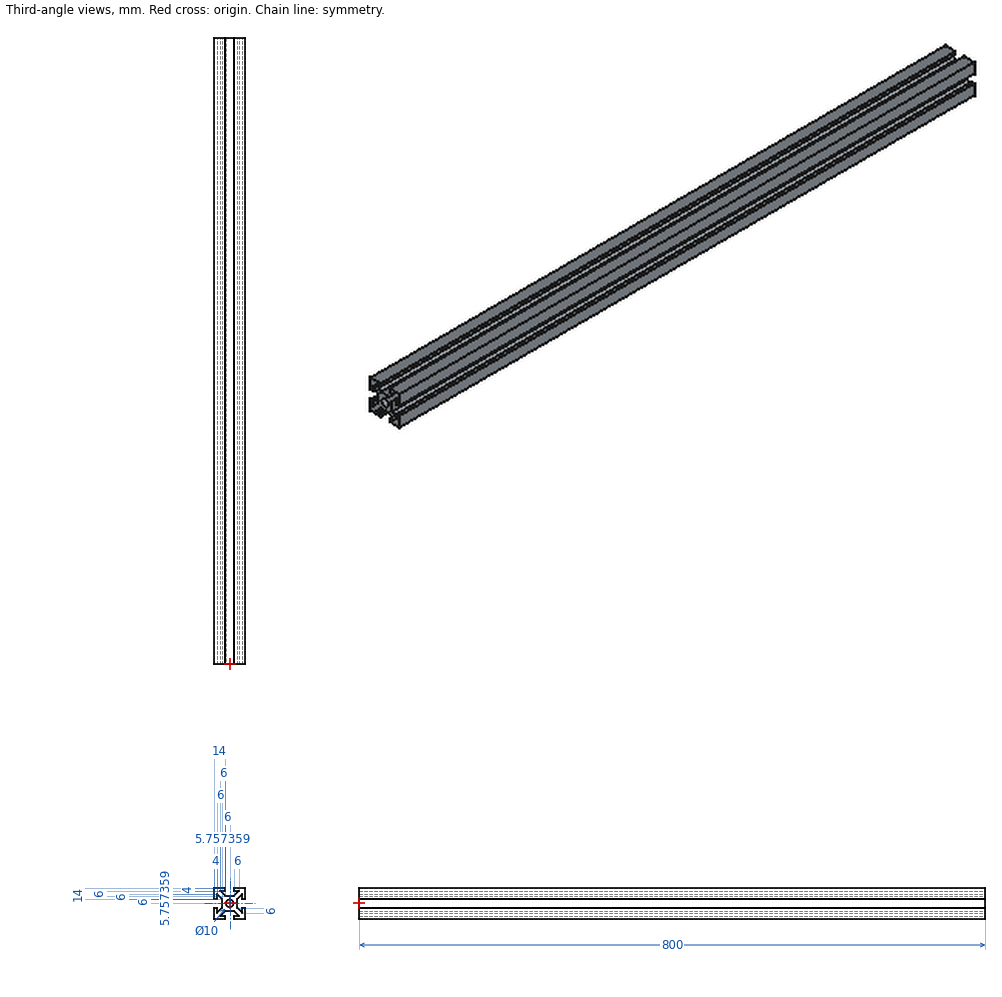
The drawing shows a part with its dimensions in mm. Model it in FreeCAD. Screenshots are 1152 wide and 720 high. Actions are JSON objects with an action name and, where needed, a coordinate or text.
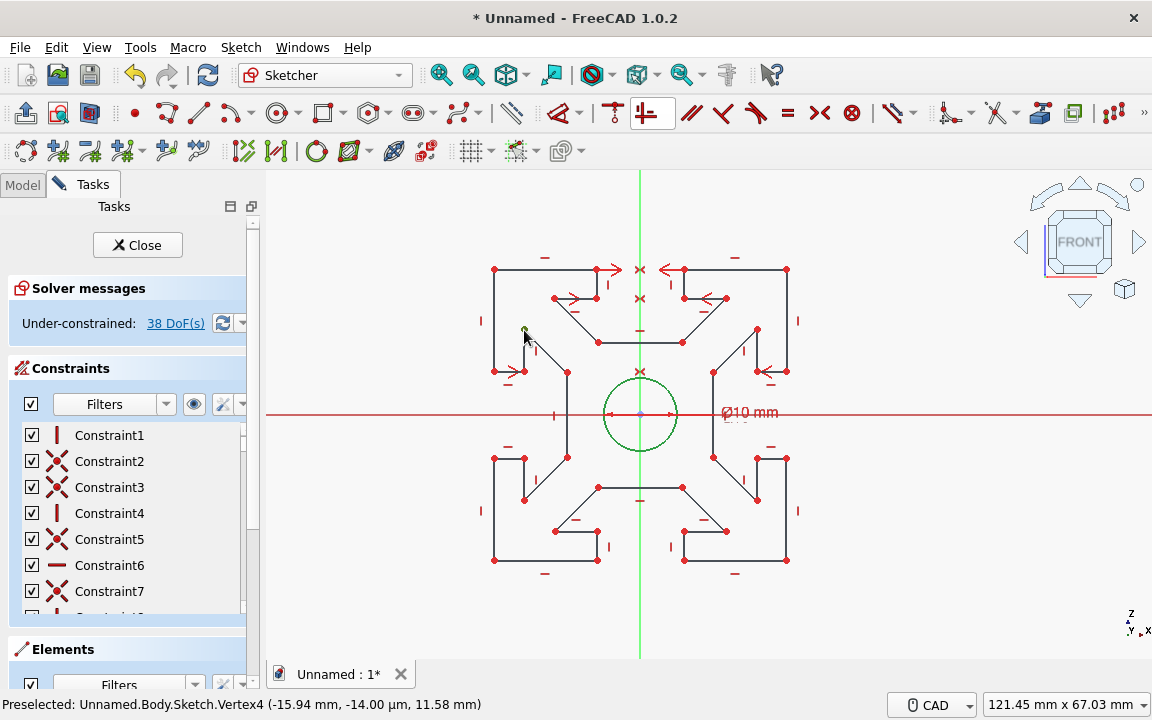
{"action": "left_click", "coordinate": [757, 330]}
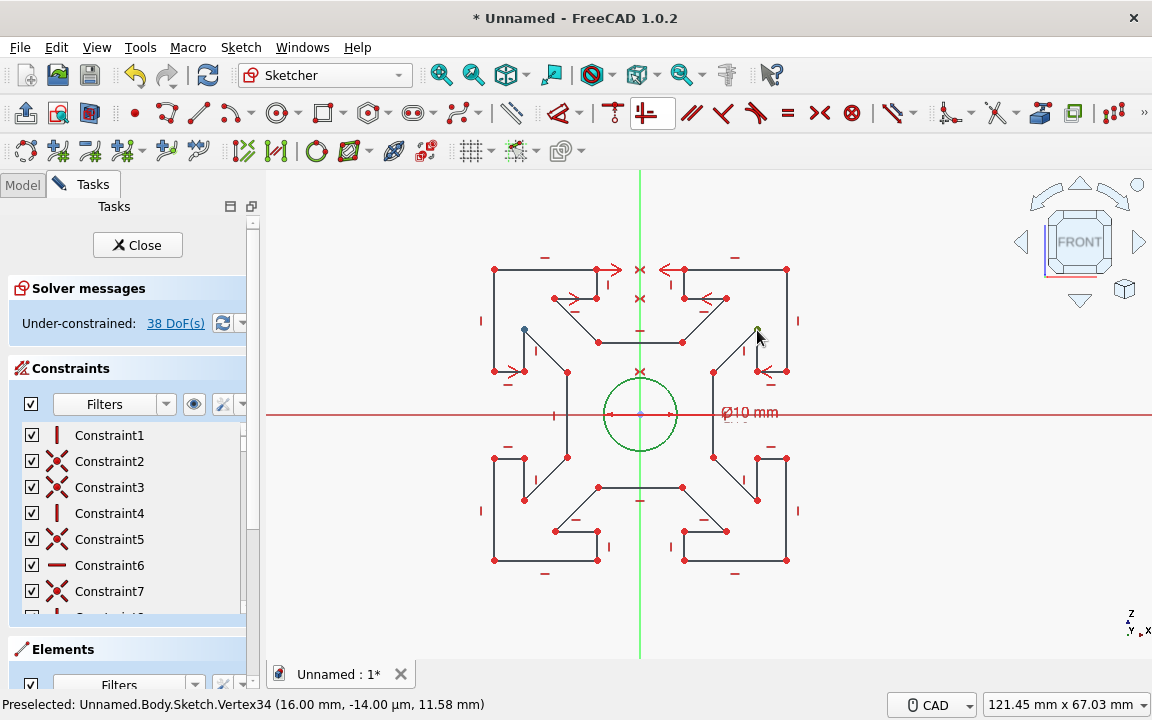
{"action": "left_click", "coordinate": [640, 600]}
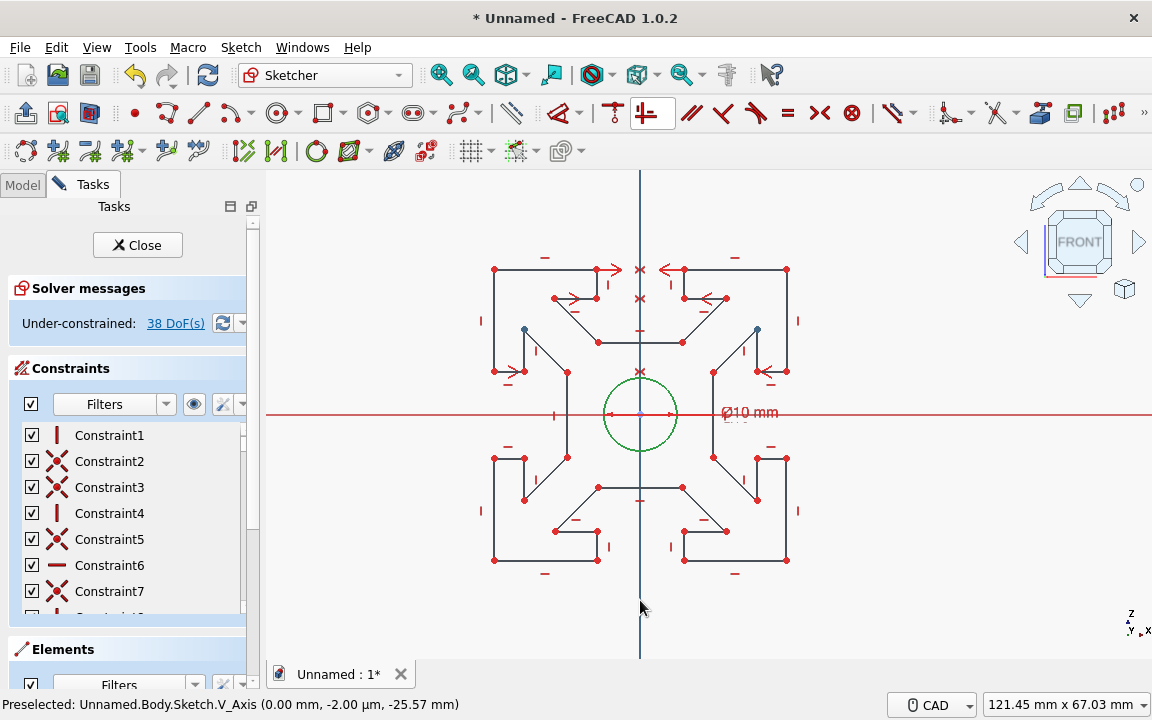
{"action": "key", "text": "s"}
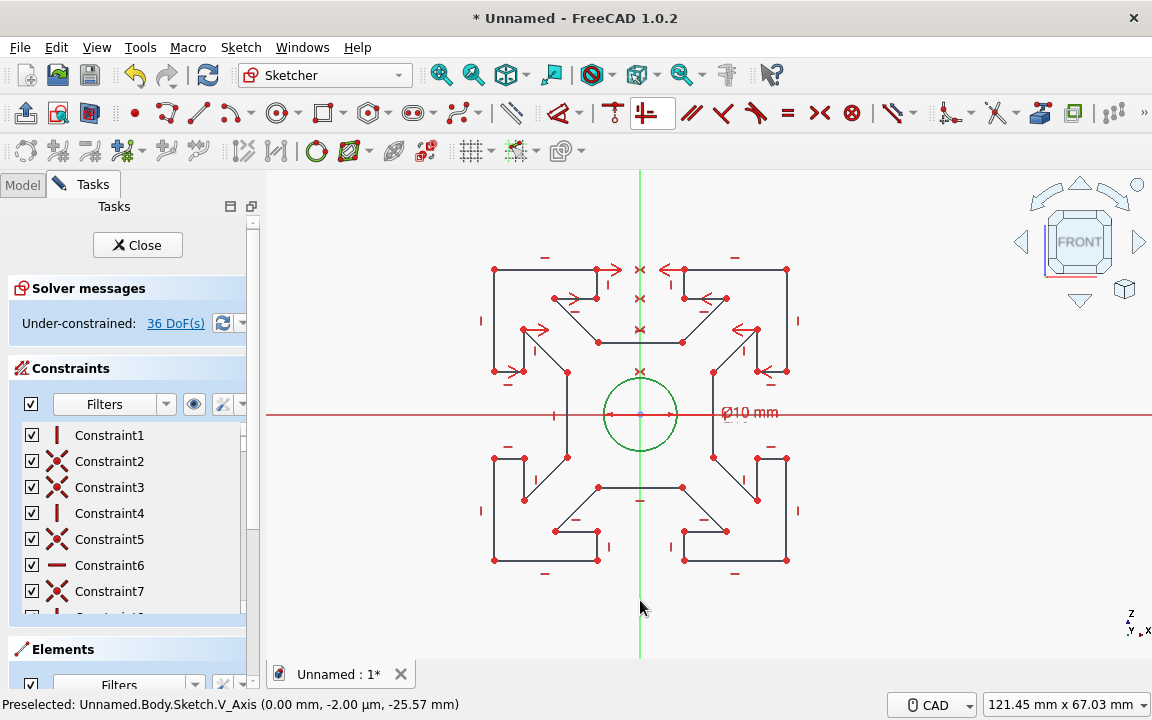
{"action": "left_click", "coordinate": [567, 373]}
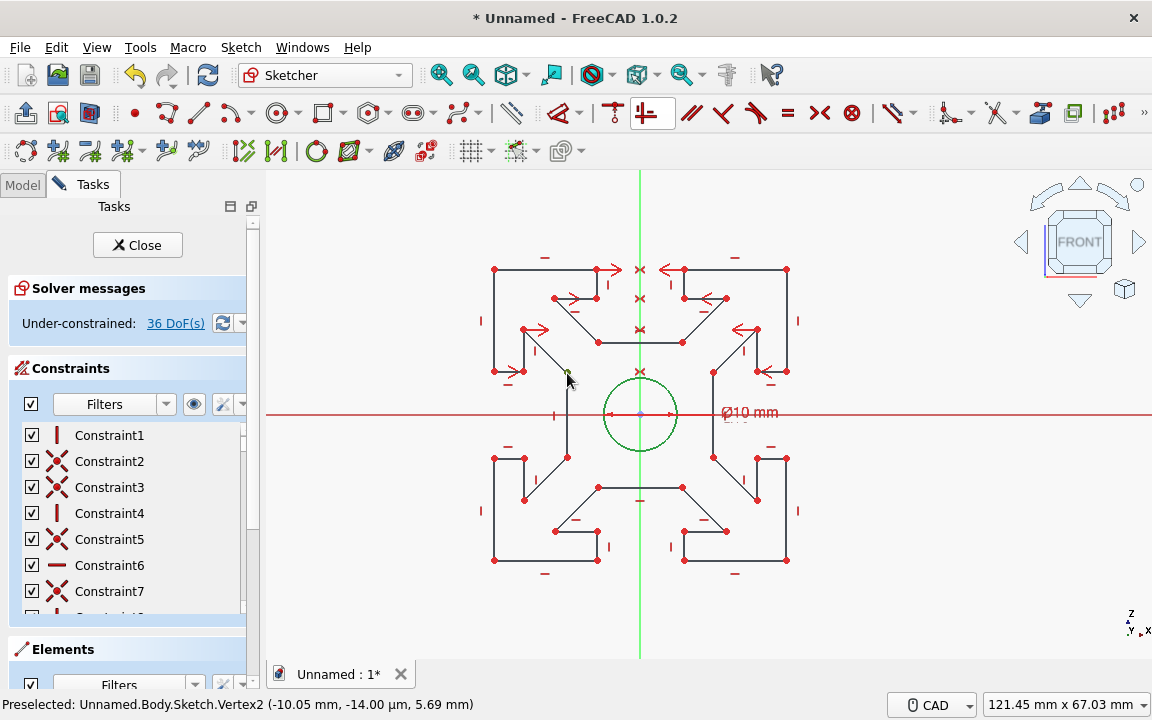
{"action": "left_click", "coordinate": [713, 373]}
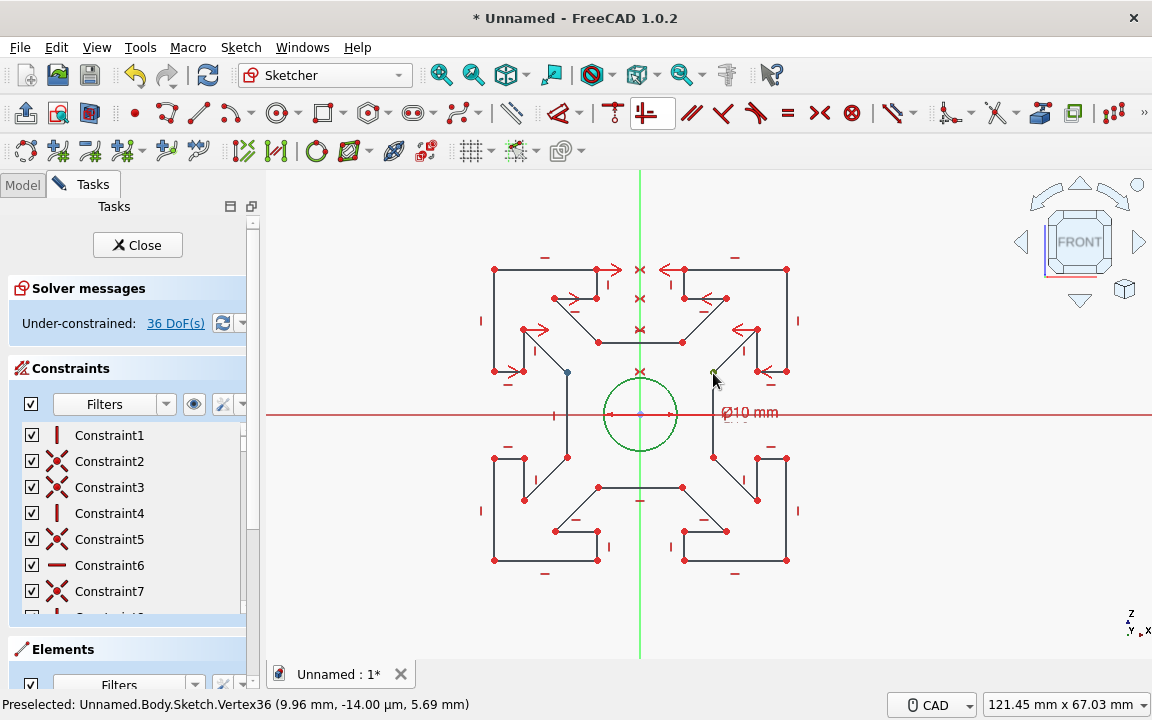
{"action": "left_click", "coordinate": [640, 600]}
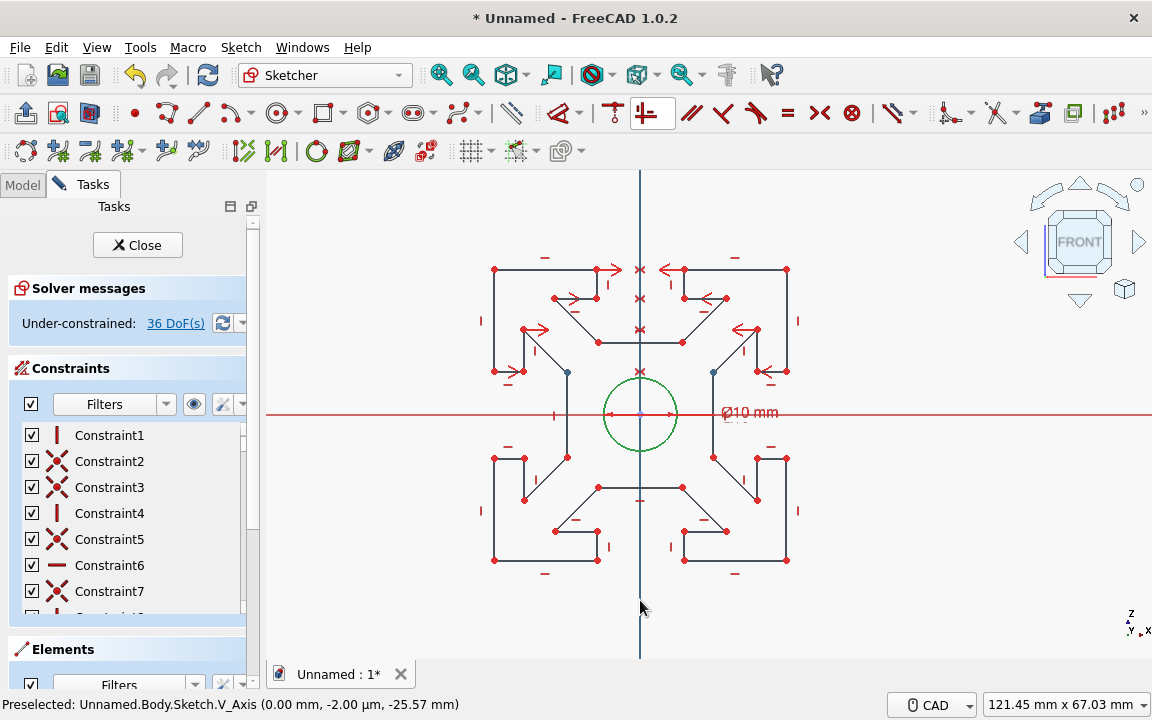
{"action": "left_click", "coordinate": [820, 114]}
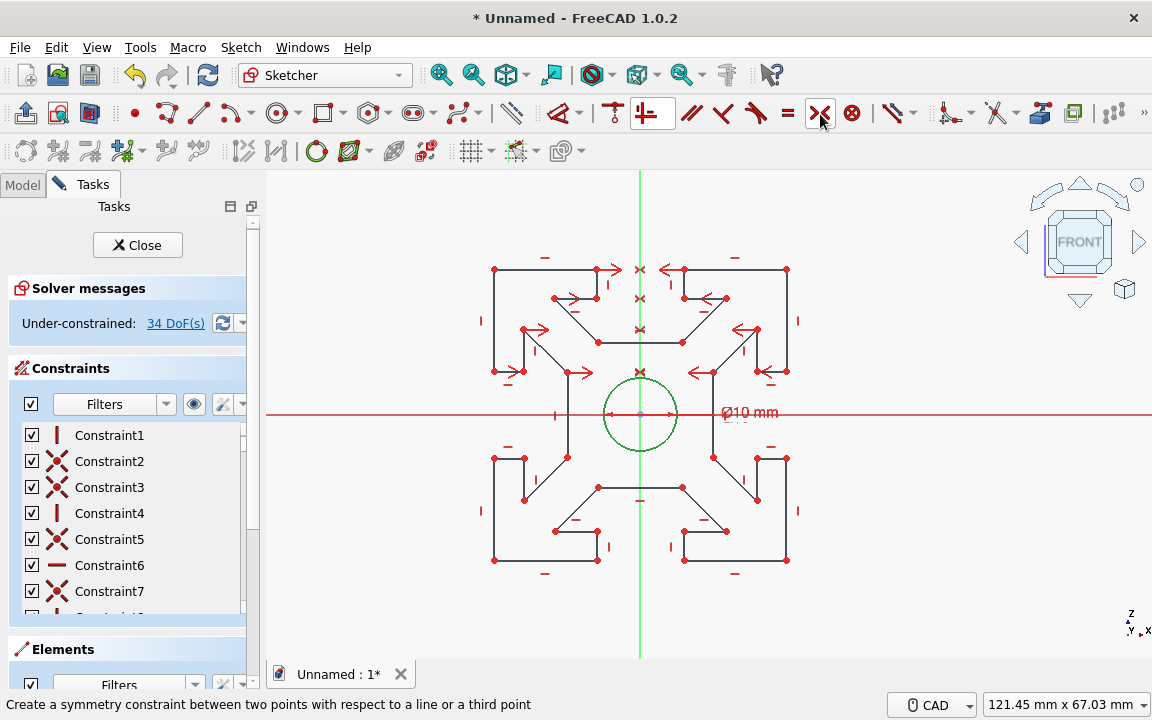
{"action": "left_click", "coordinate": [757, 330]}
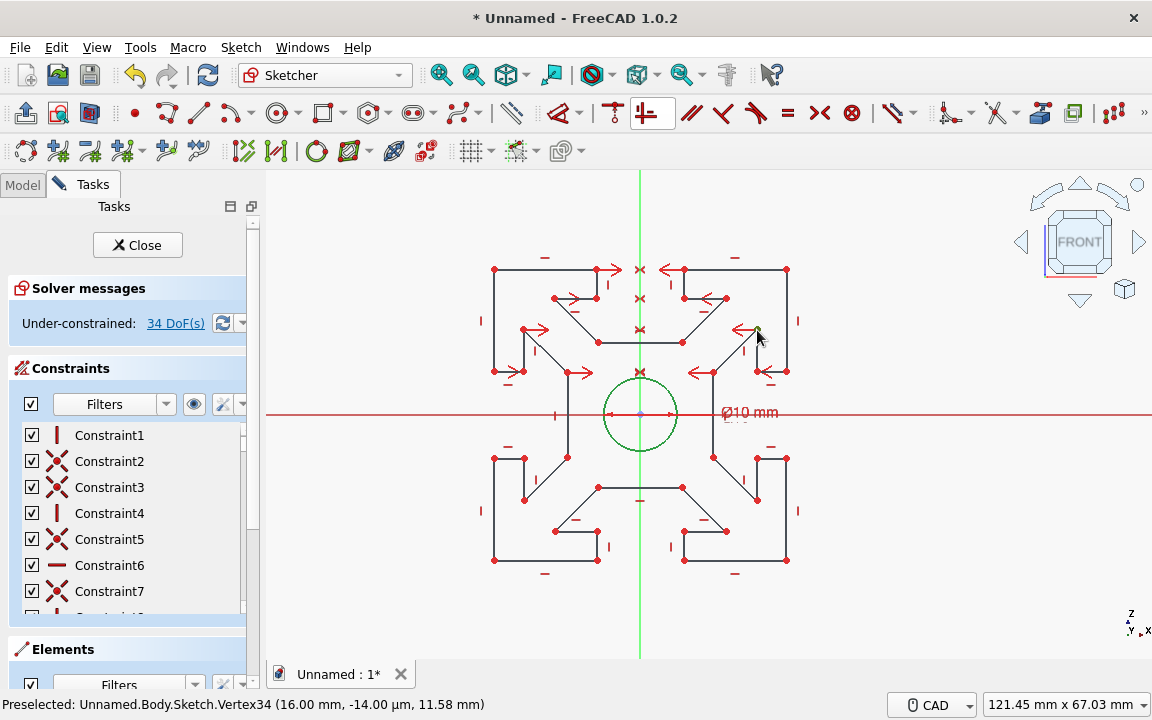
{"action": "left_click", "coordinate": [757, 501]}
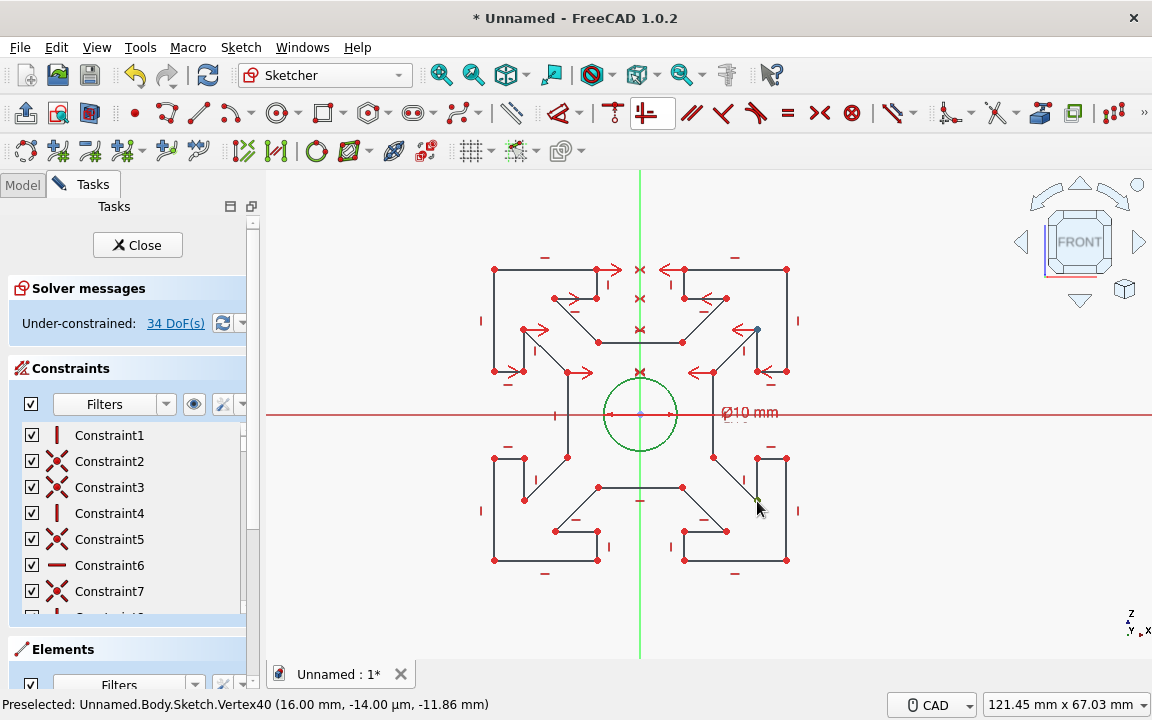
{"action": "left_click", "coordinate": [344, 414]}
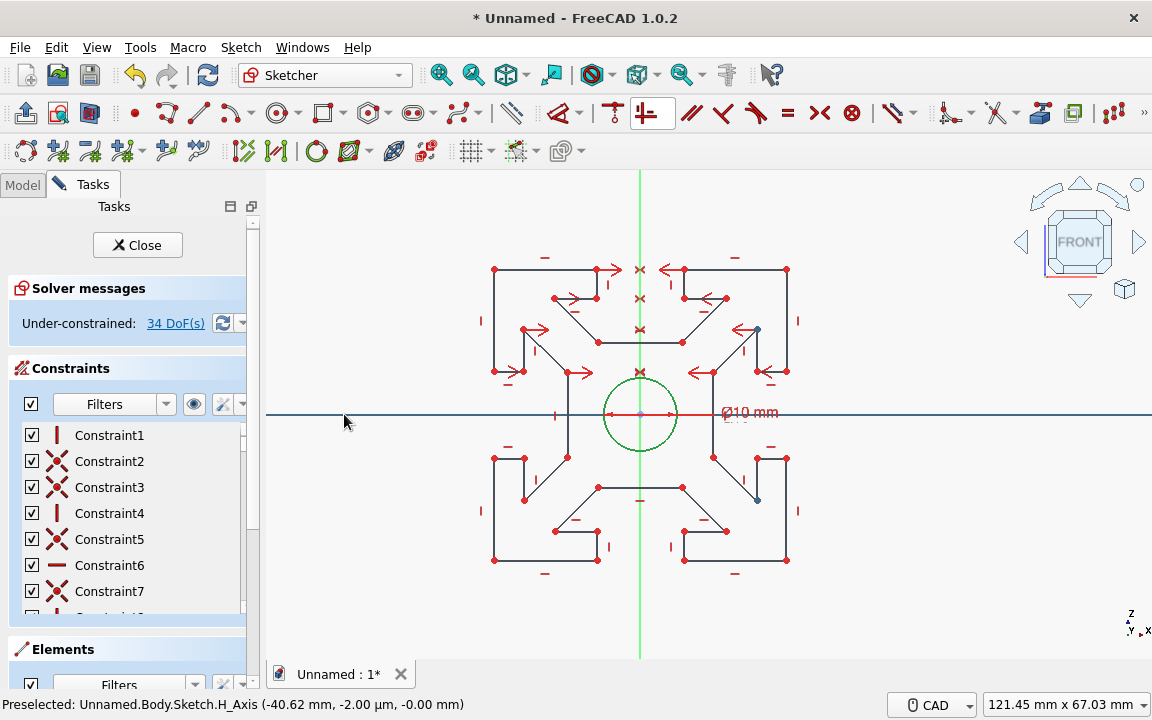
{"action": "key", "text": "s"}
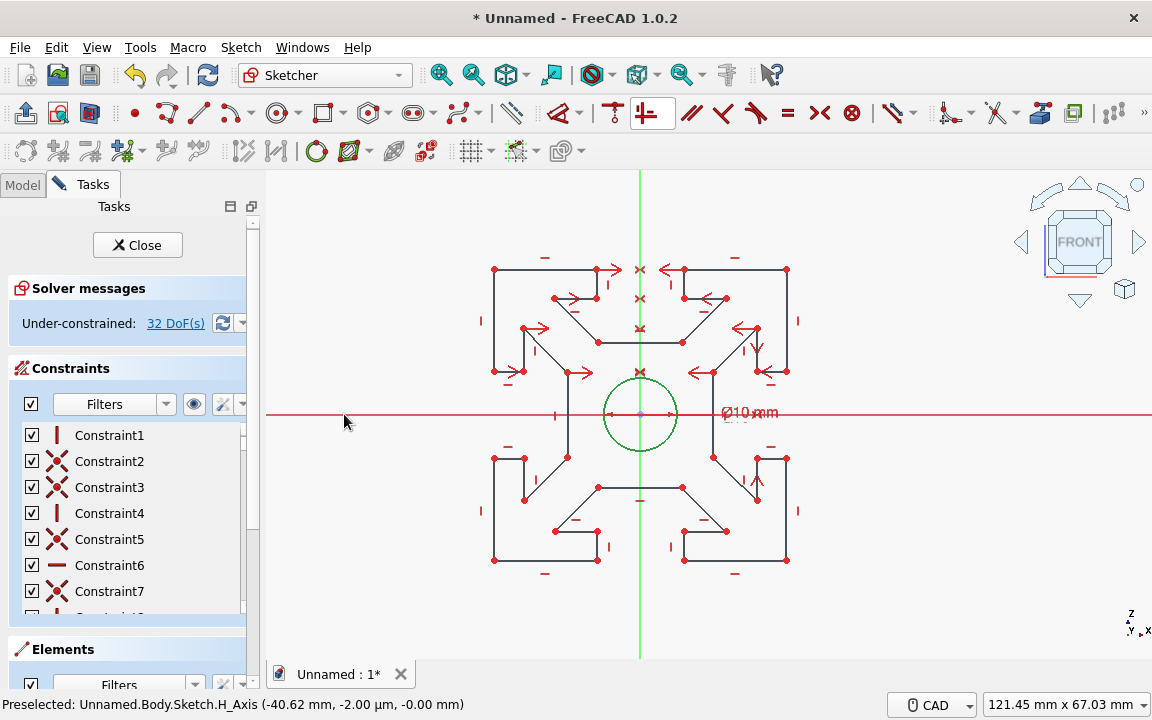
{"action": "left_click", "coordinate": [787, 372]}